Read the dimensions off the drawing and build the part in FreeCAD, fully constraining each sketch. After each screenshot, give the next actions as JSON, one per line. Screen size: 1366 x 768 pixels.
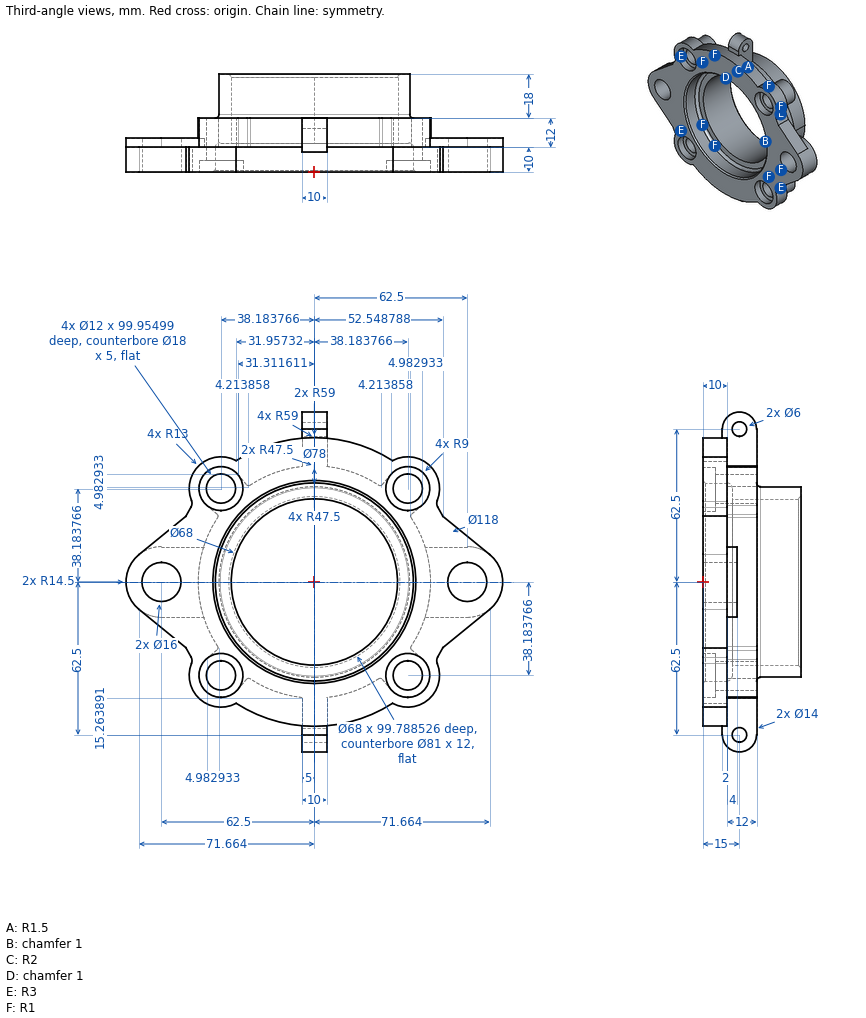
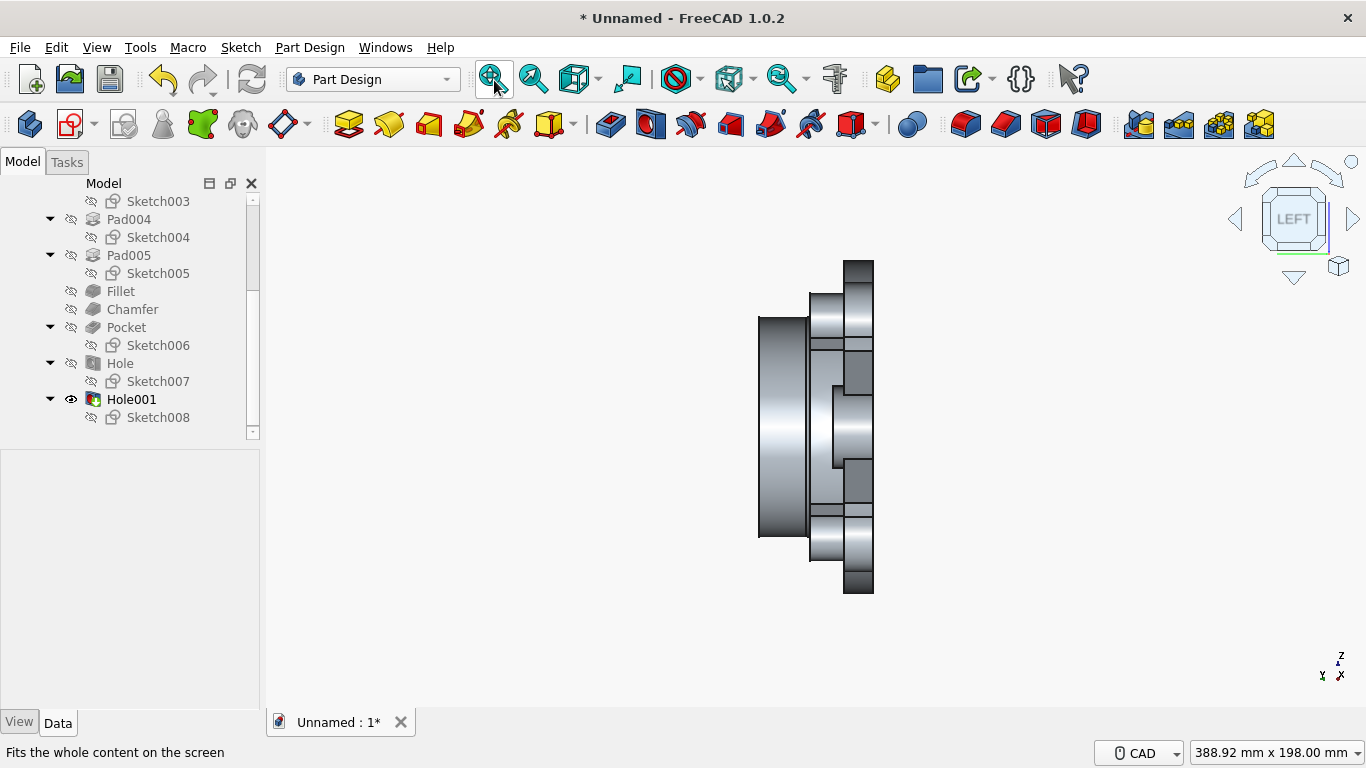
{"action": "key", "text": "v 3"}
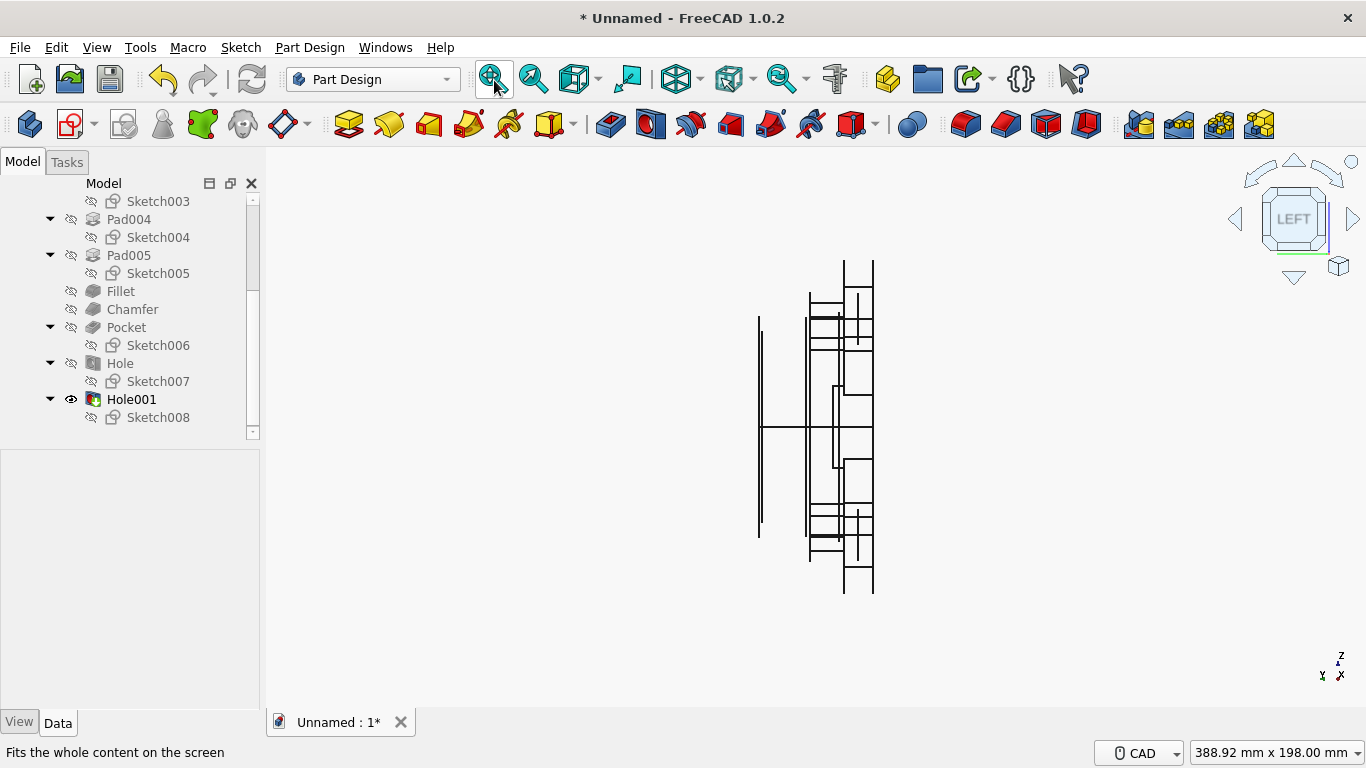
{"action": "key", "text": "0"}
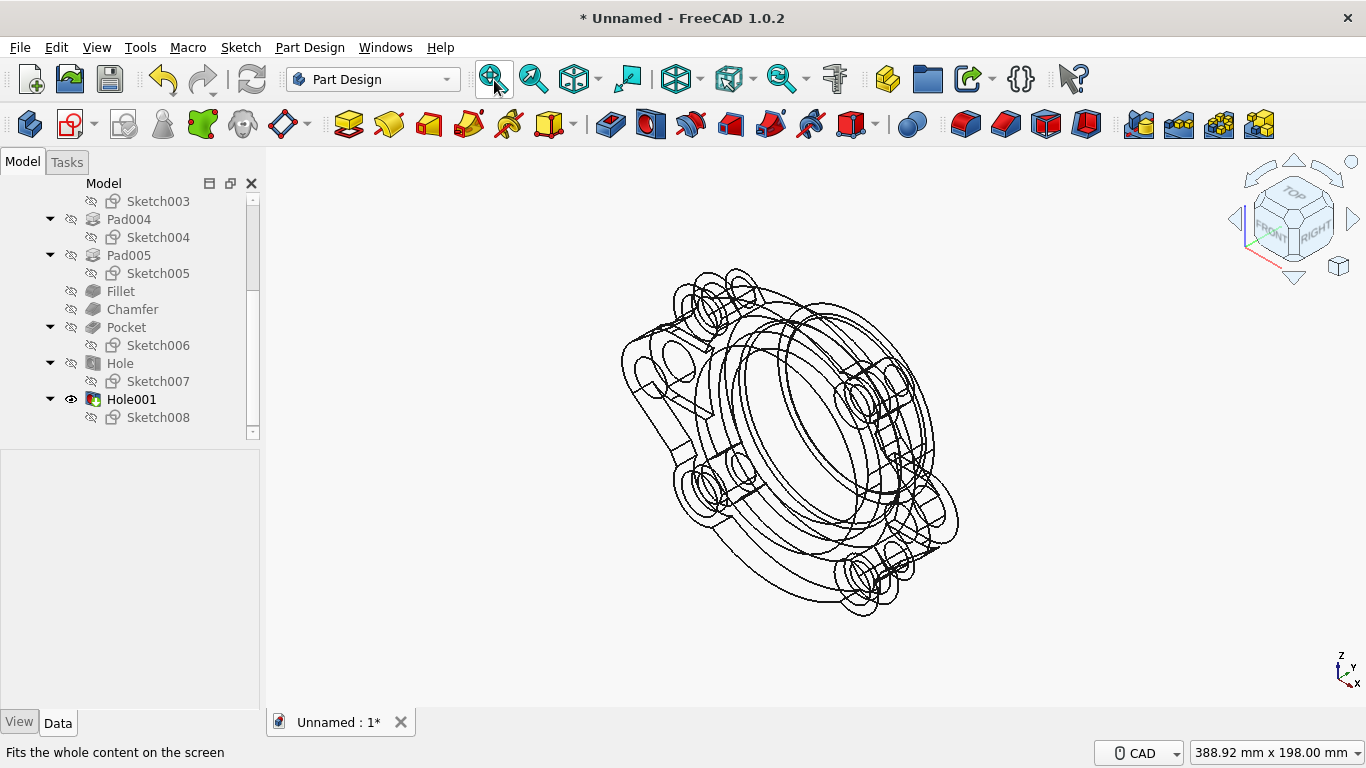
{"action": "left_click", "coordinate": [719, 388]}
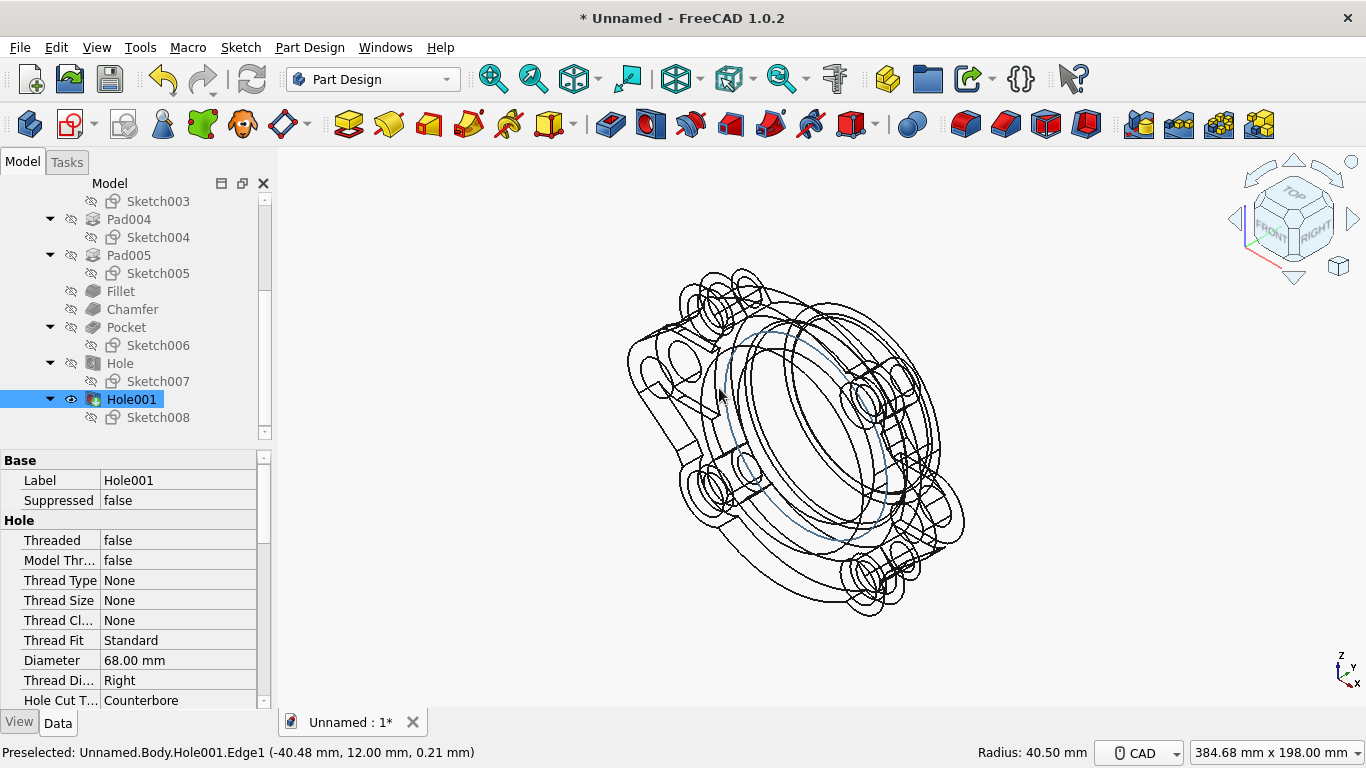
{"action": "key", "text": "v 1"}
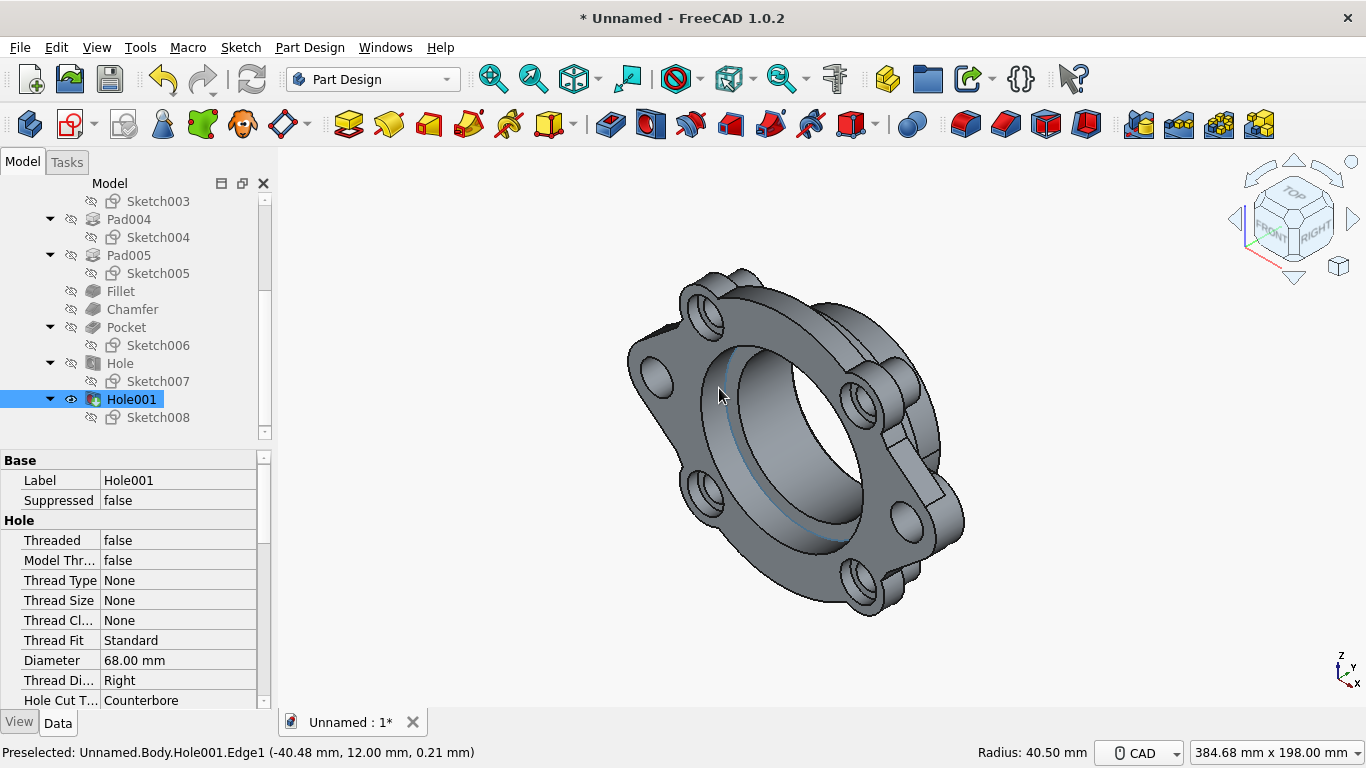
{"action": "left_click", "coordinate": [966, 124]}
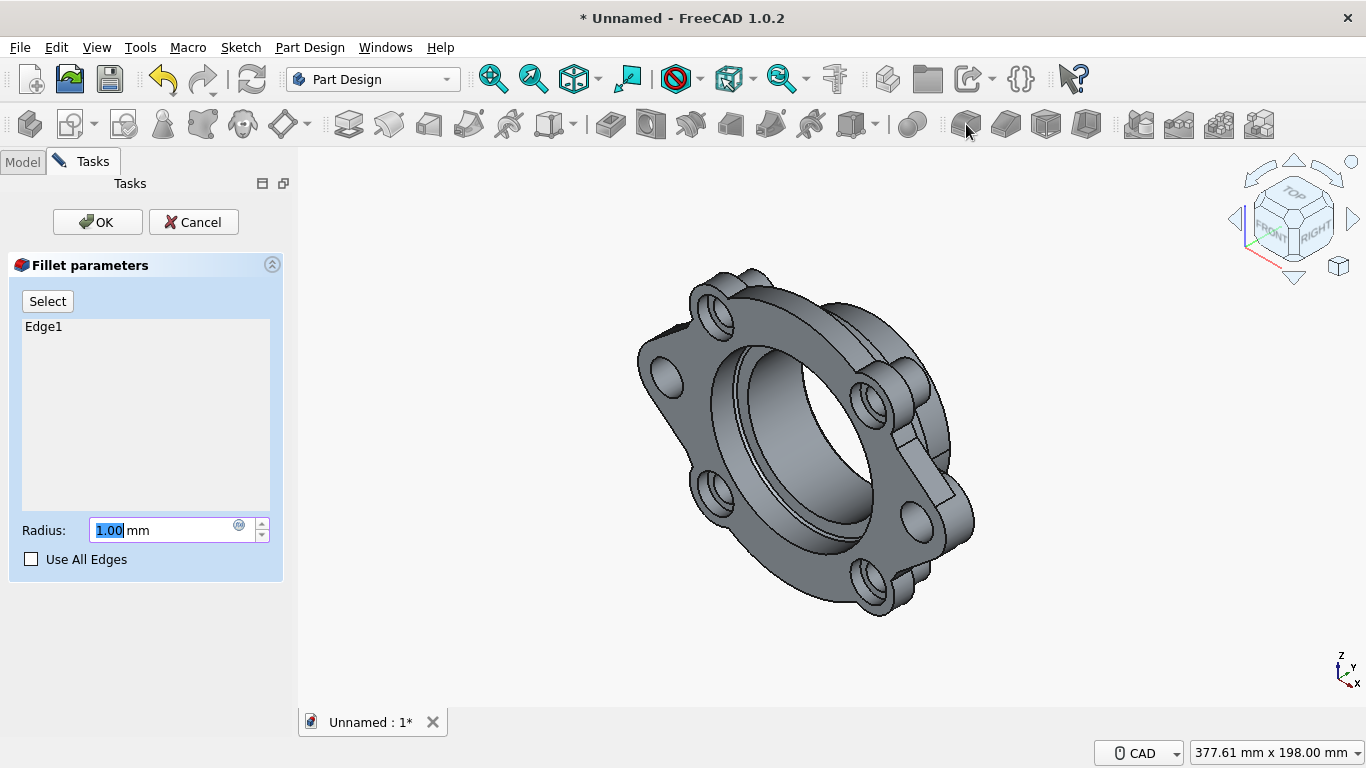
{"action": "type", "text": "2"}
{"action": "key", "text": "Tab"}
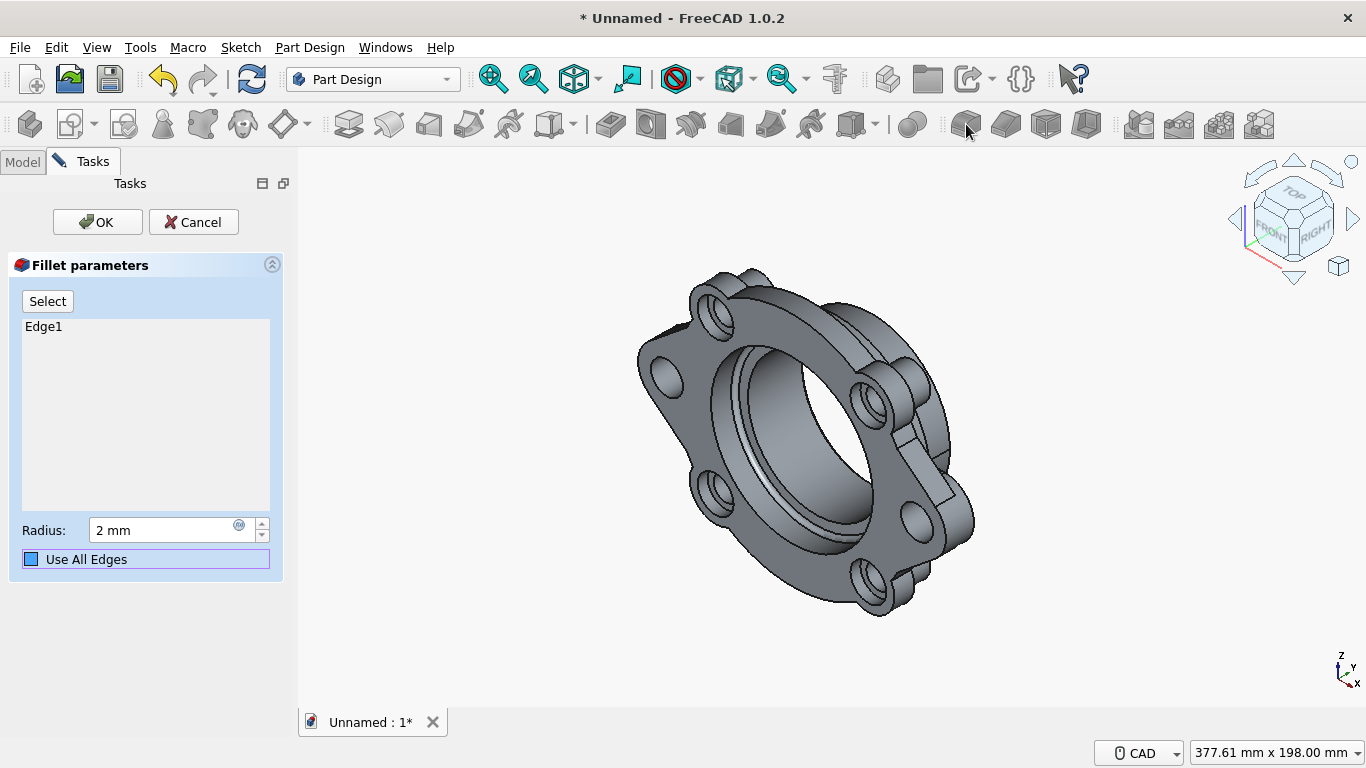
{"action": "left_click", "coordinate": [98, 222]}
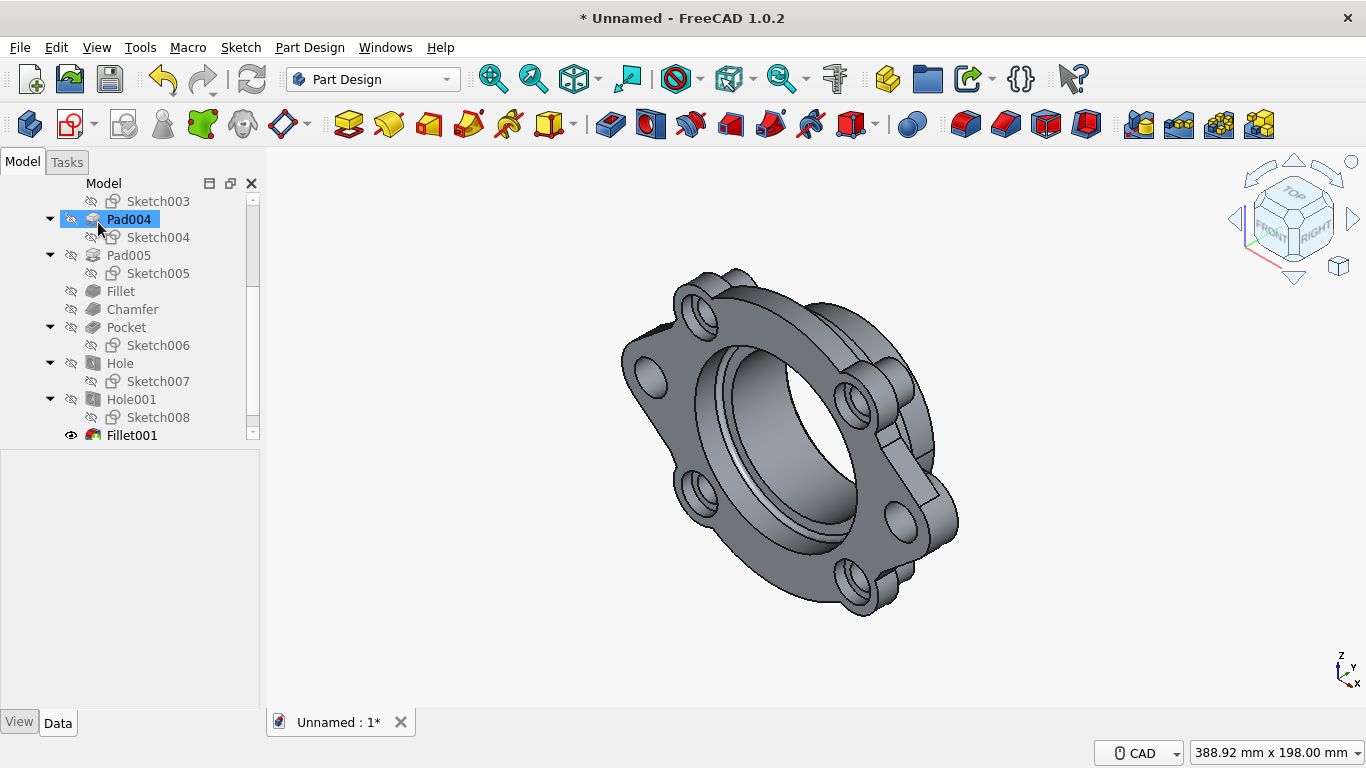
{"action": "left_click", "coordinate": [695, 402]}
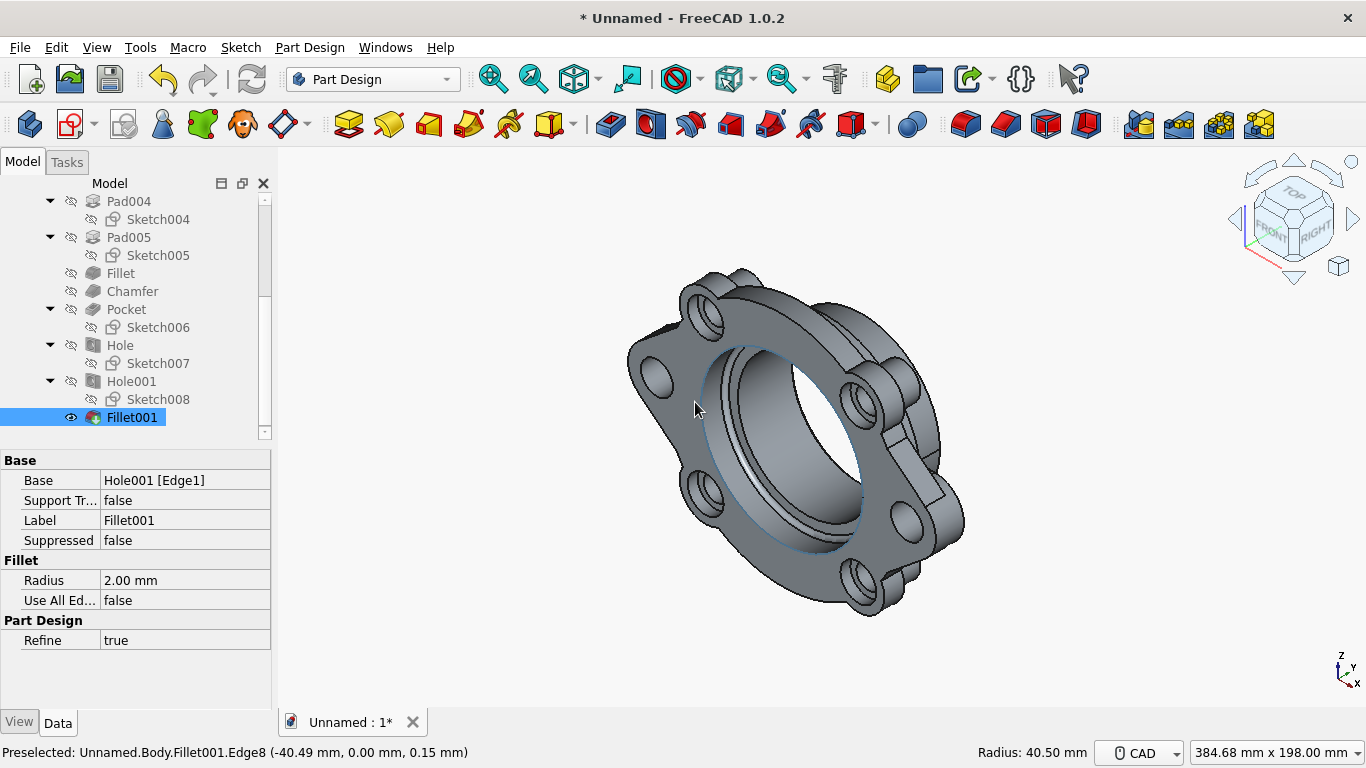
{"action": "left_click", "coordinate": [1006, 124]}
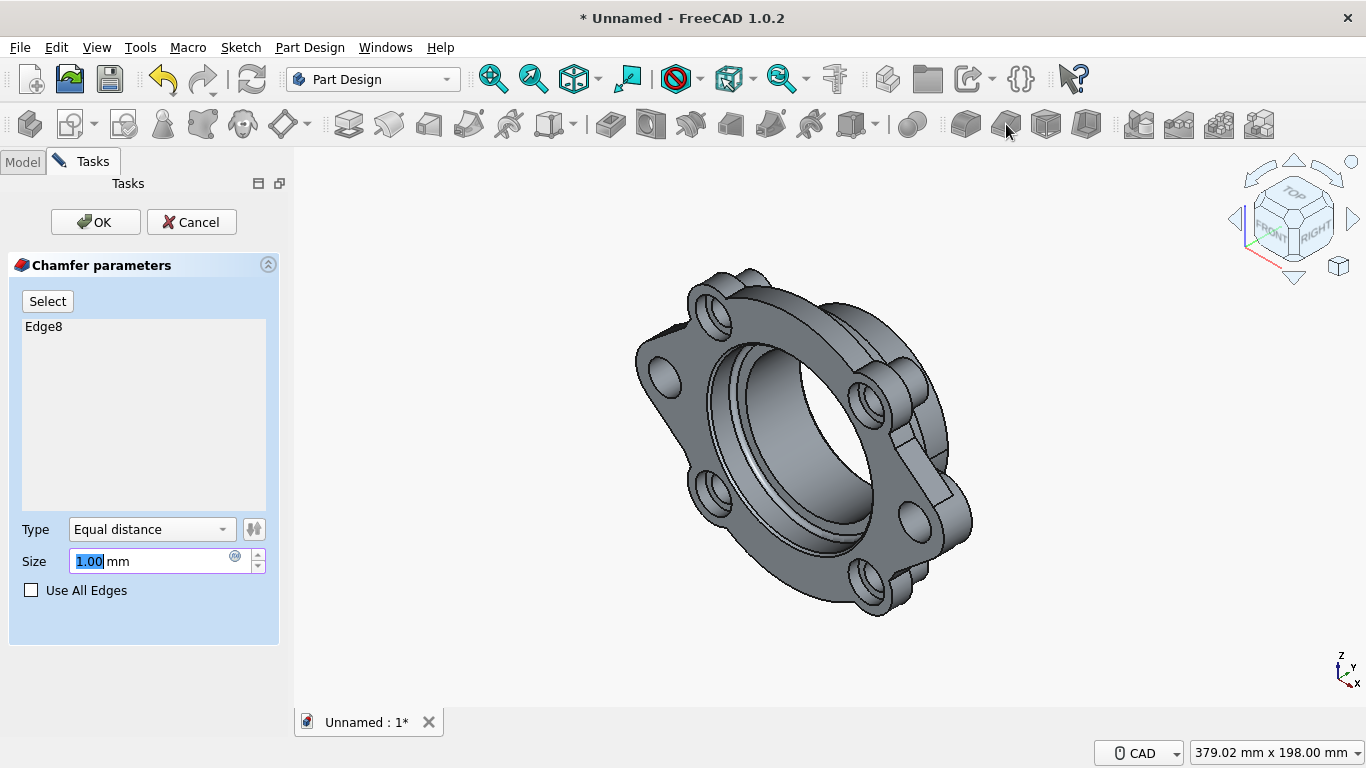
{"action": "type", "text": "1"}
{"action": "key", "text": "Tab"}